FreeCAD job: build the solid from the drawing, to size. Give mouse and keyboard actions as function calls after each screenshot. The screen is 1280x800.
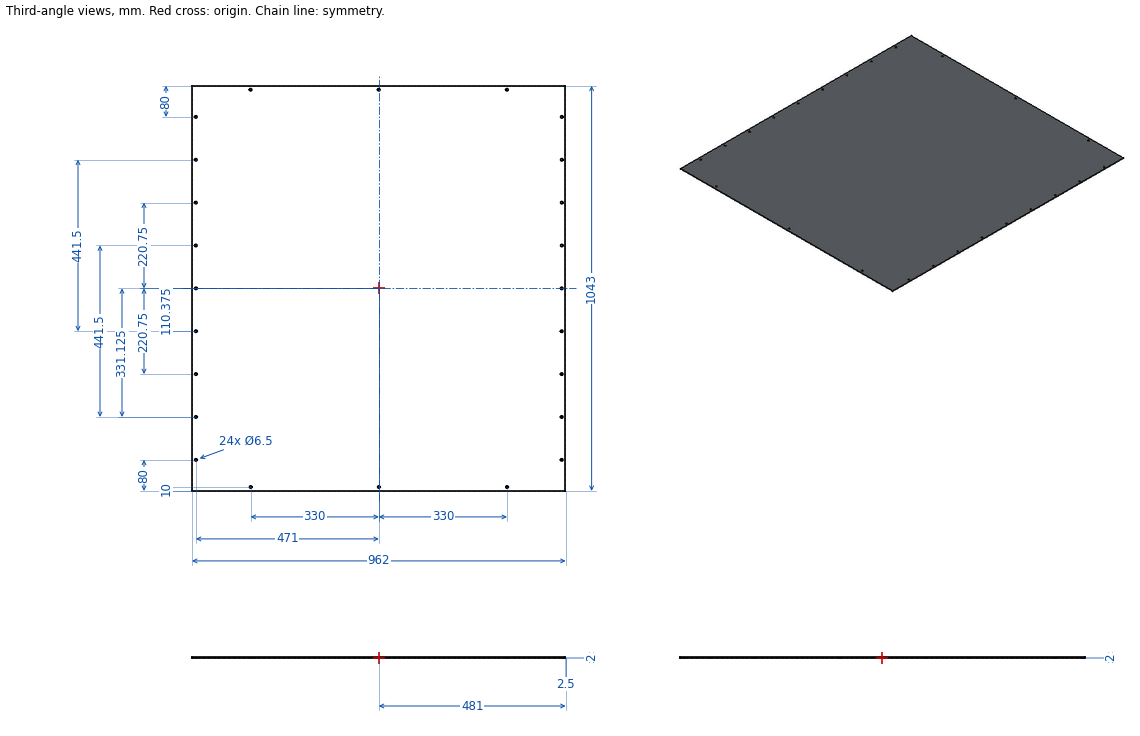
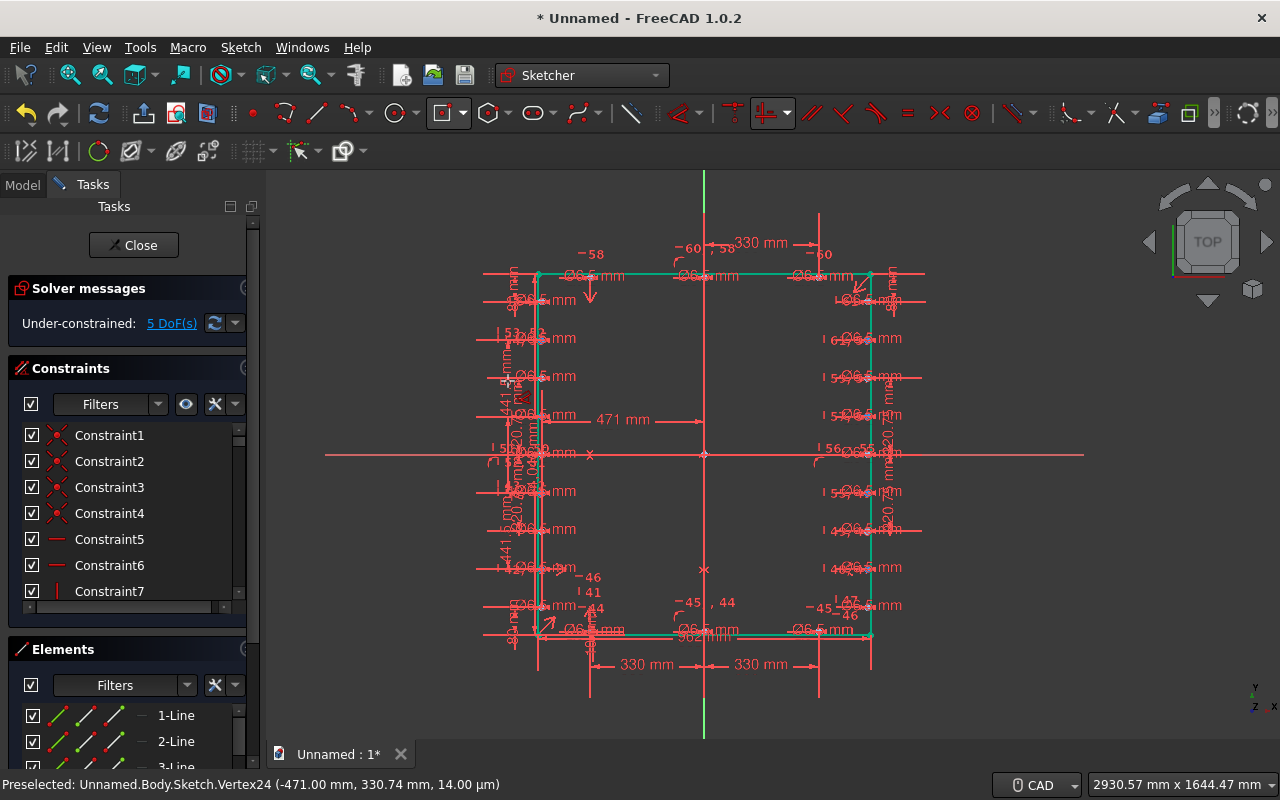
click(867, 569)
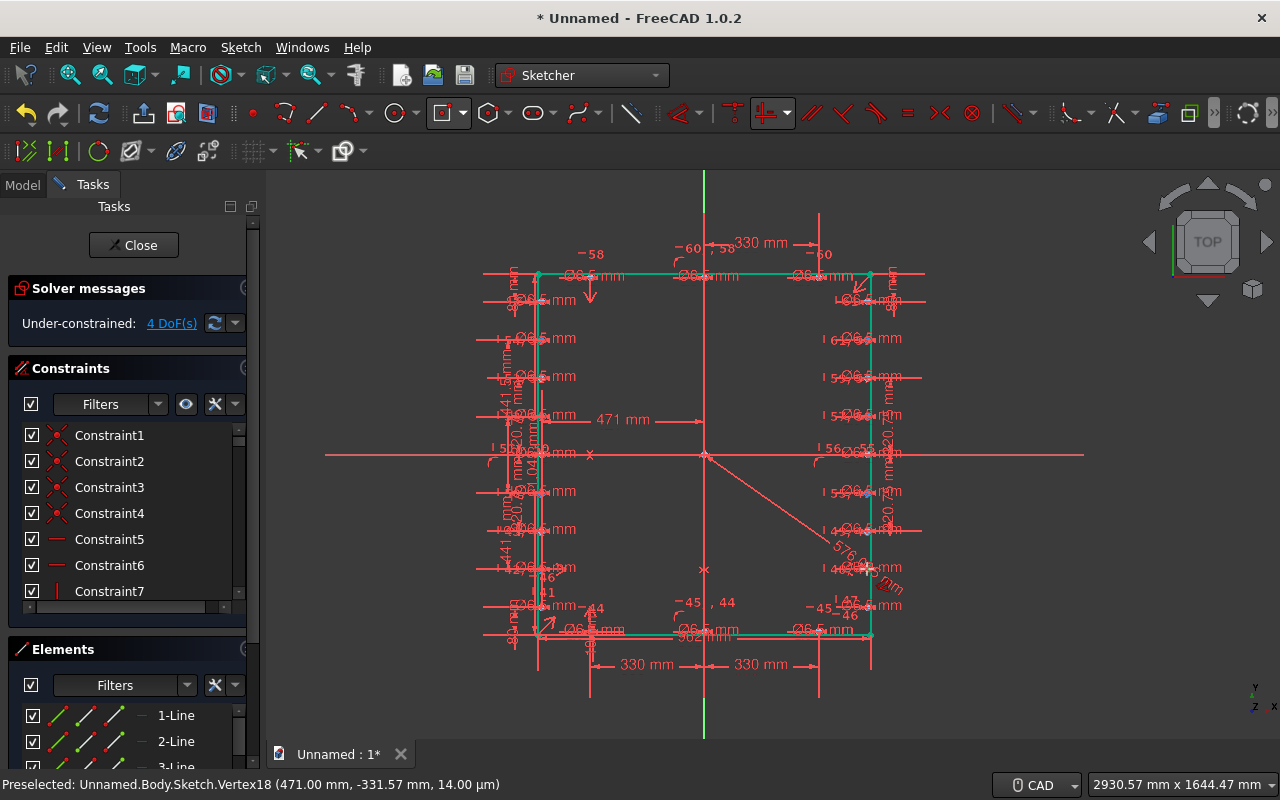
click(867, 417)
click(901, 528)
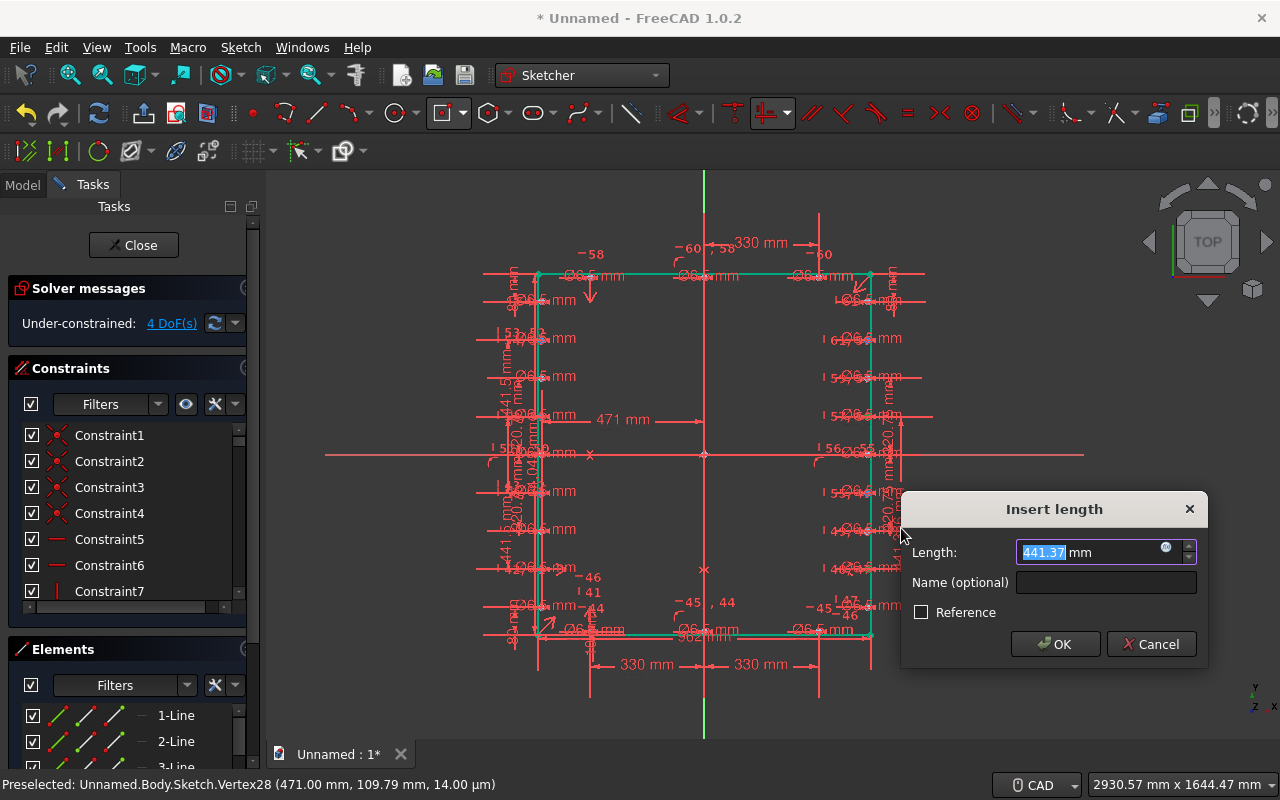
text(441.5)
key(Return)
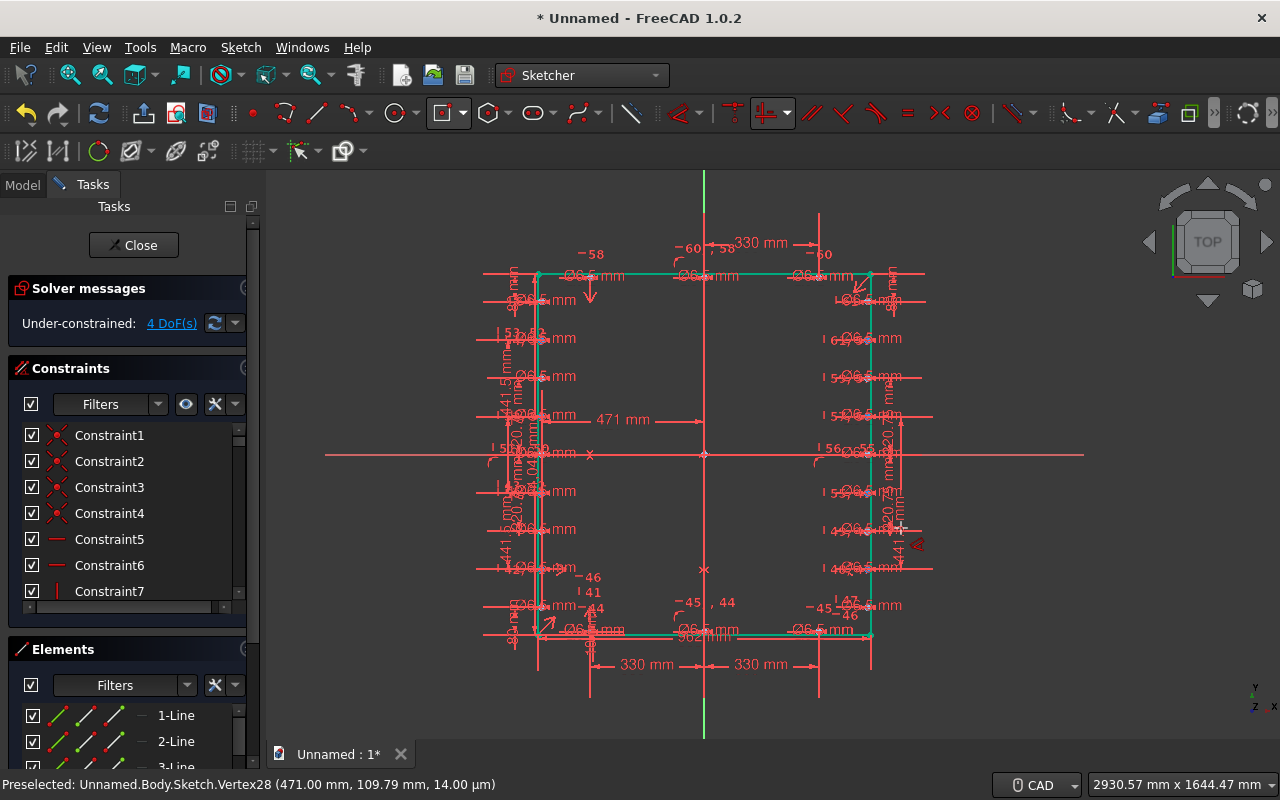
click(867, 493)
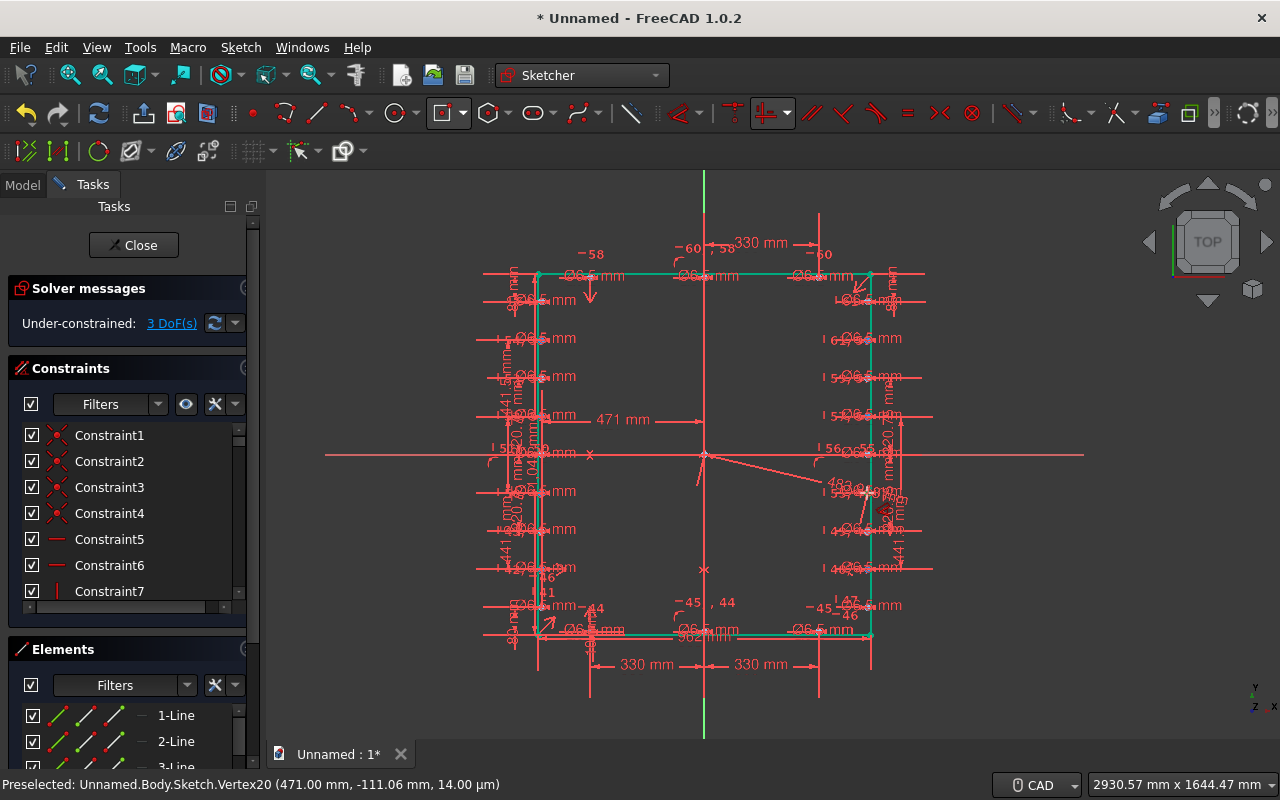
click(867, 340)
click(901, 382)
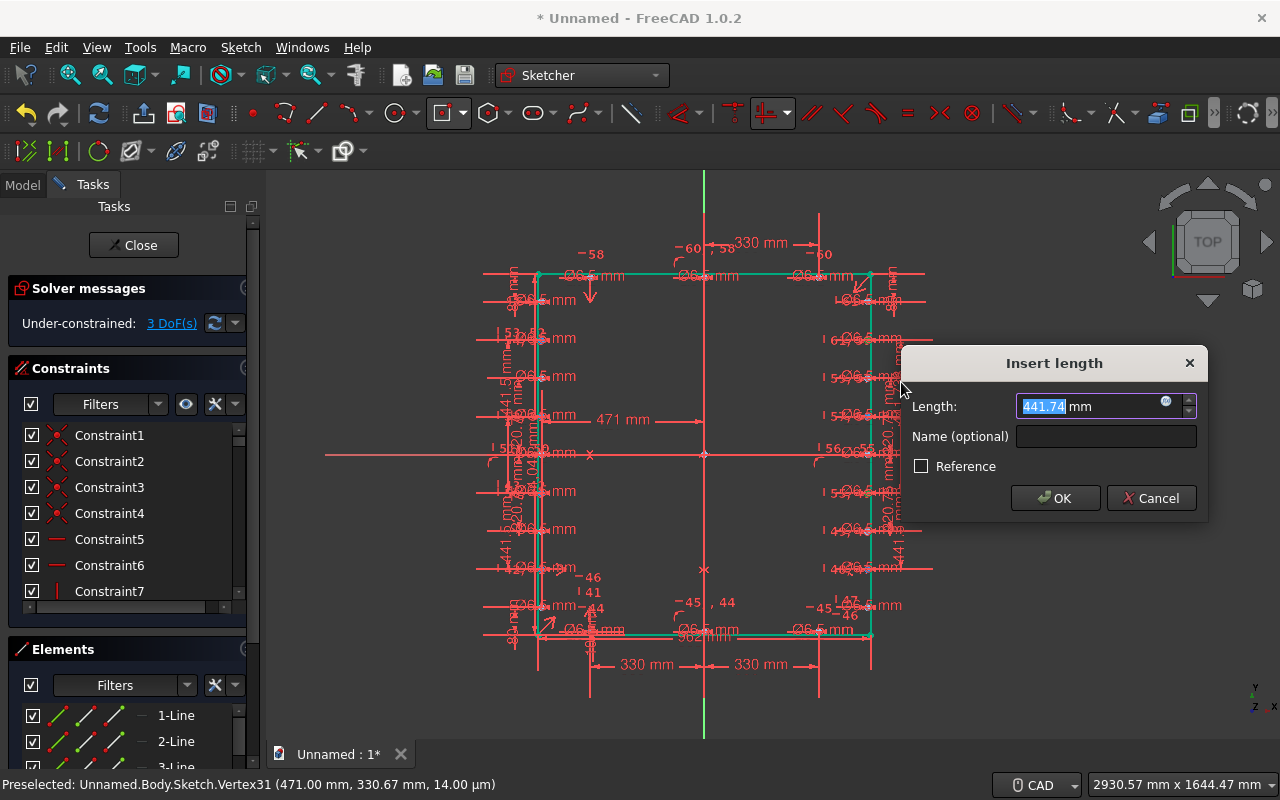
text(441.5)
key(Return)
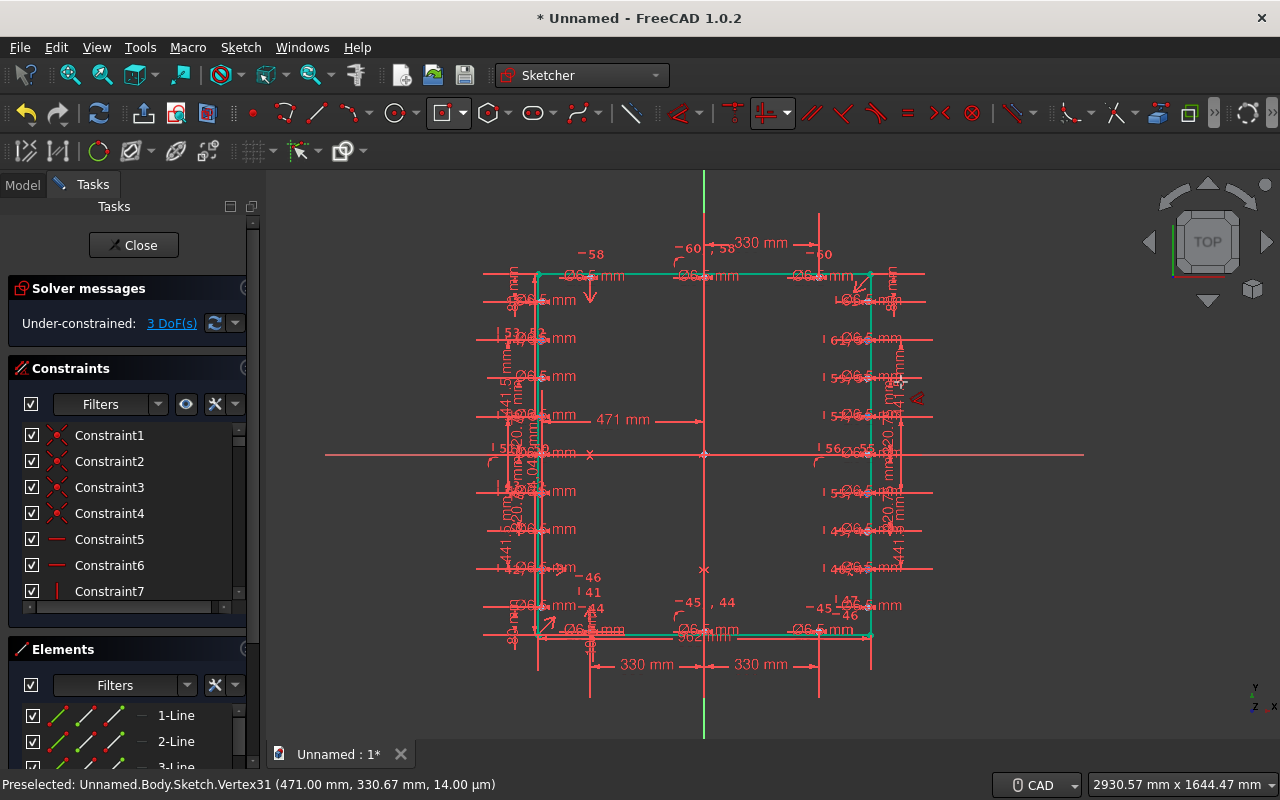
click(542, 569)
click(508, 472)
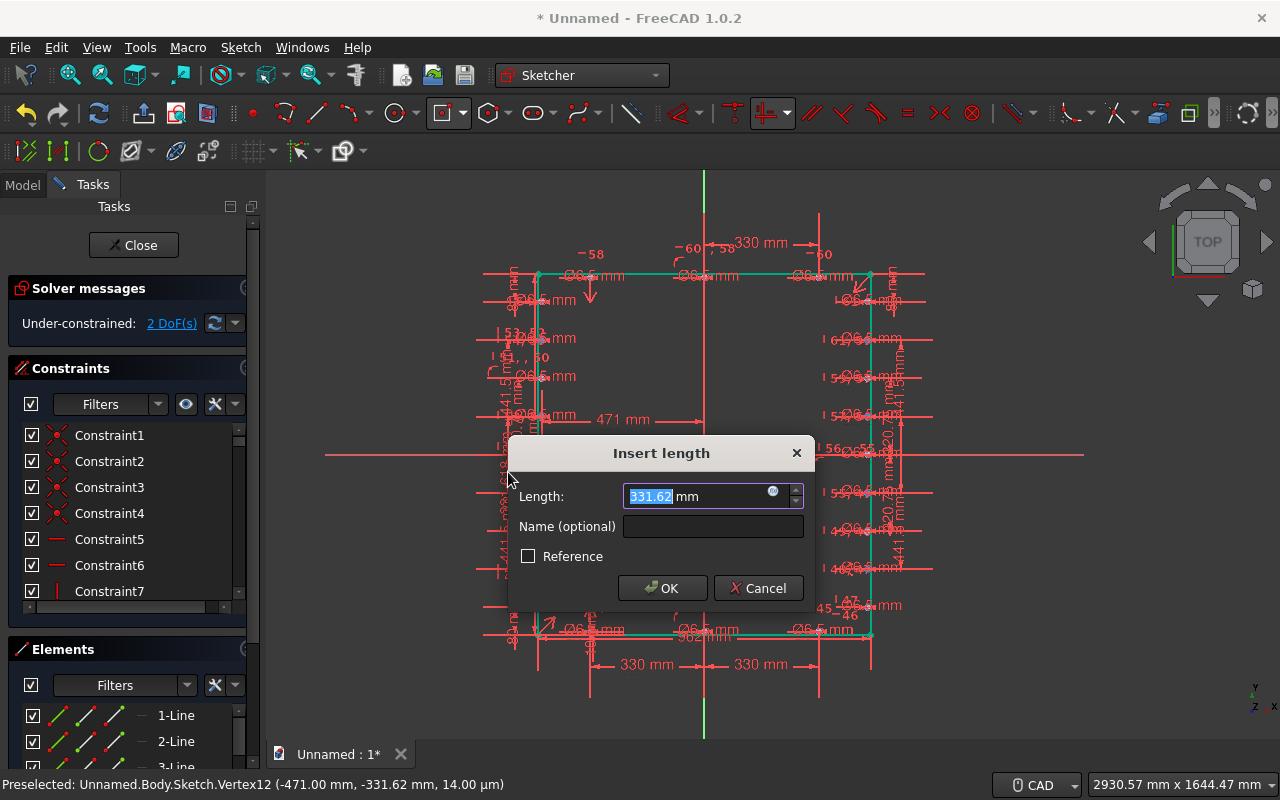
text(331.125)
key(Return)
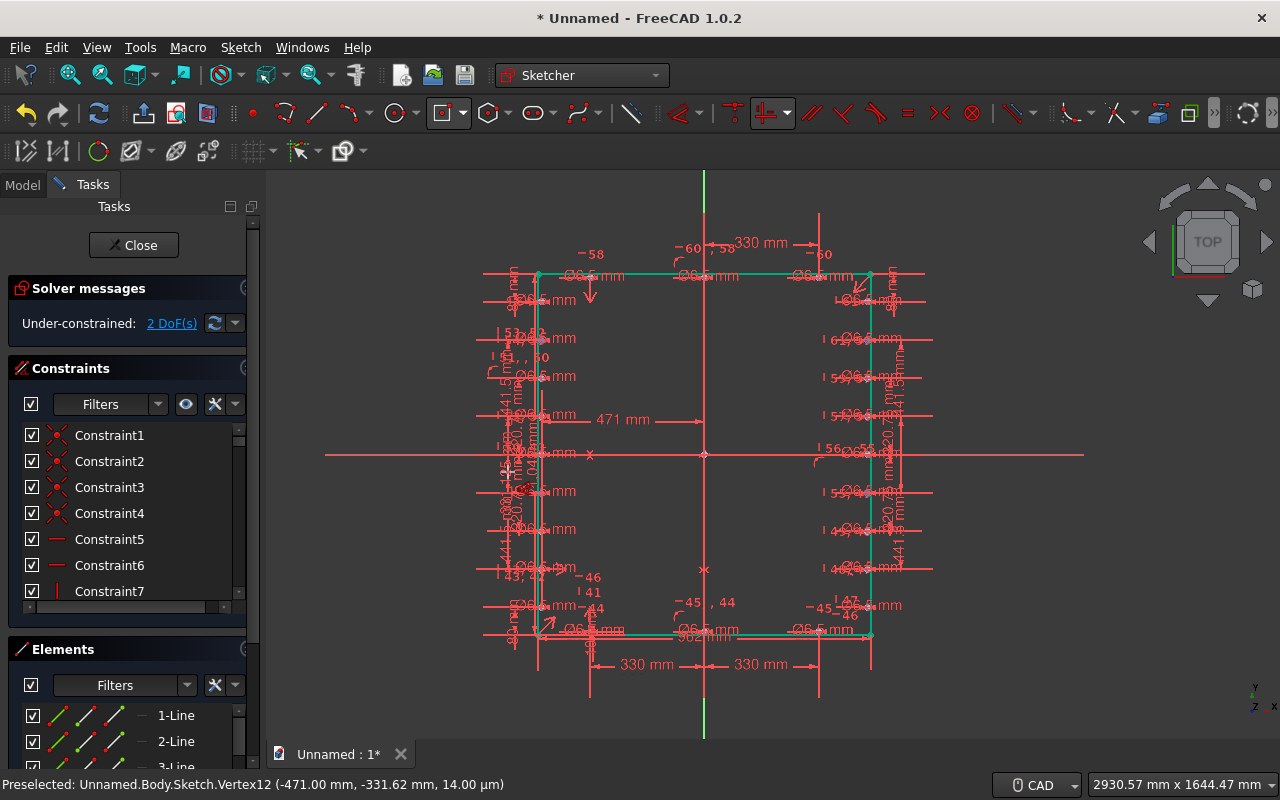
click(542, 493)
click(738, 474)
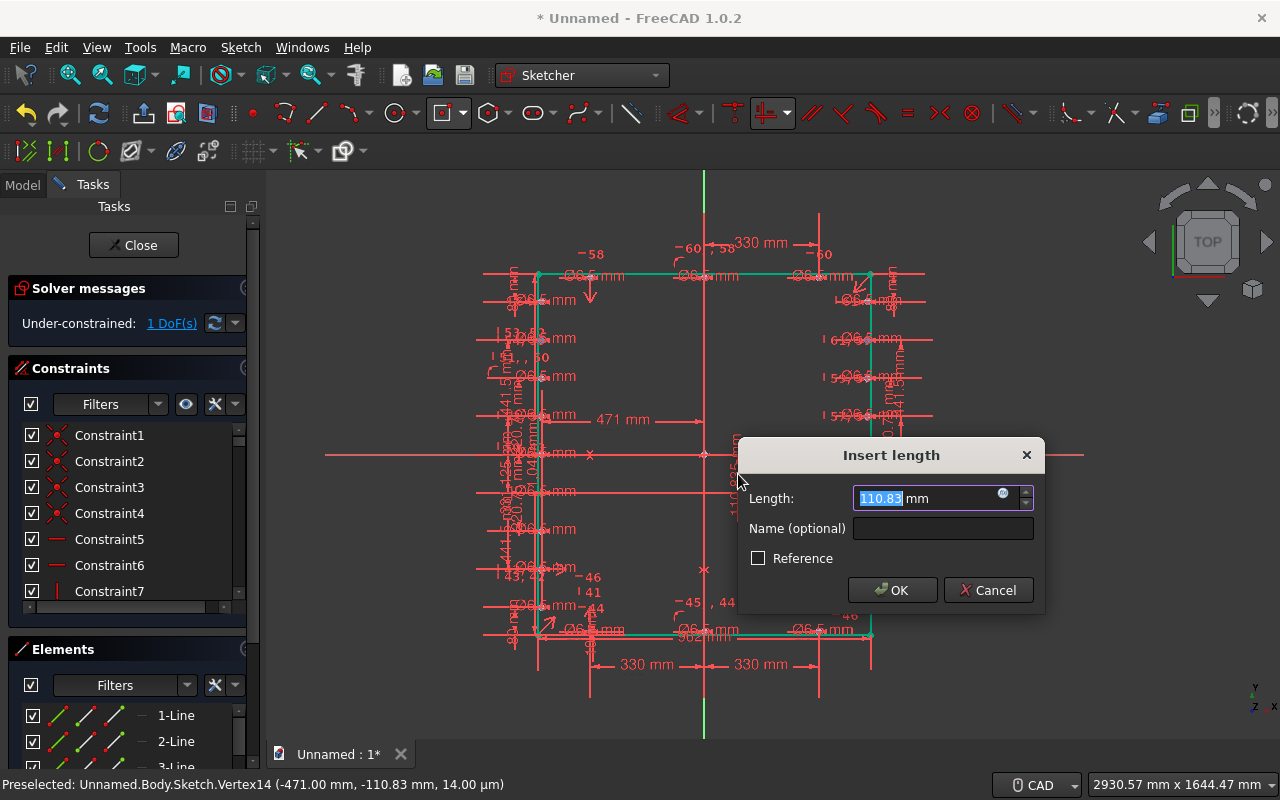
text(110.375)
key(Return)